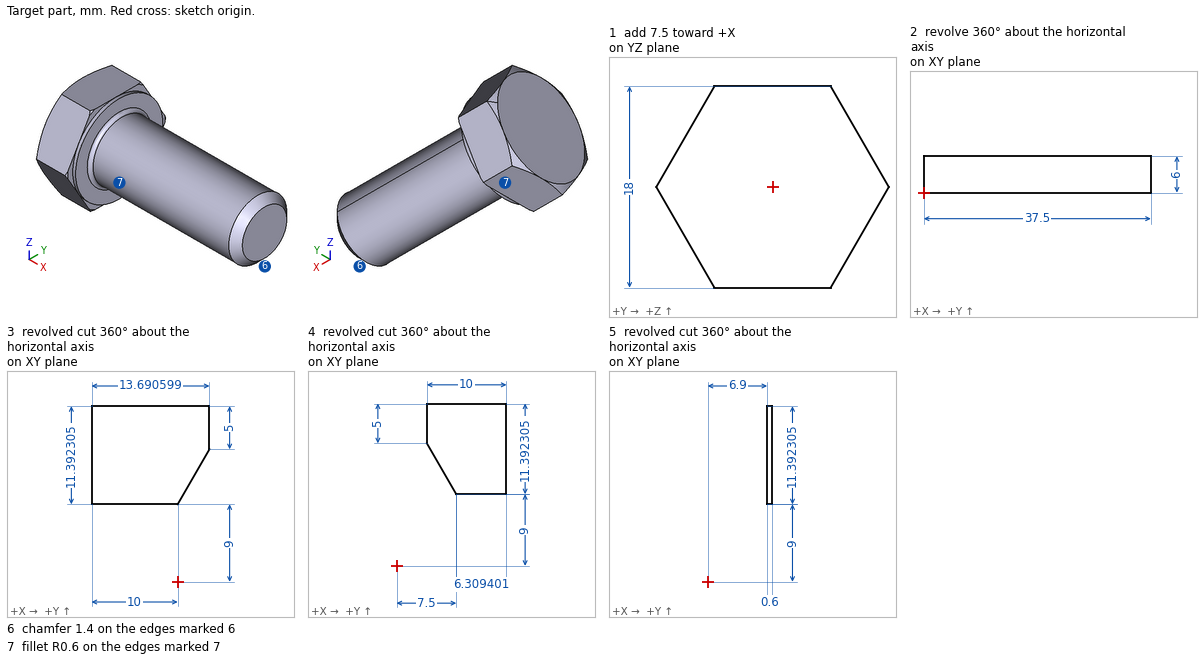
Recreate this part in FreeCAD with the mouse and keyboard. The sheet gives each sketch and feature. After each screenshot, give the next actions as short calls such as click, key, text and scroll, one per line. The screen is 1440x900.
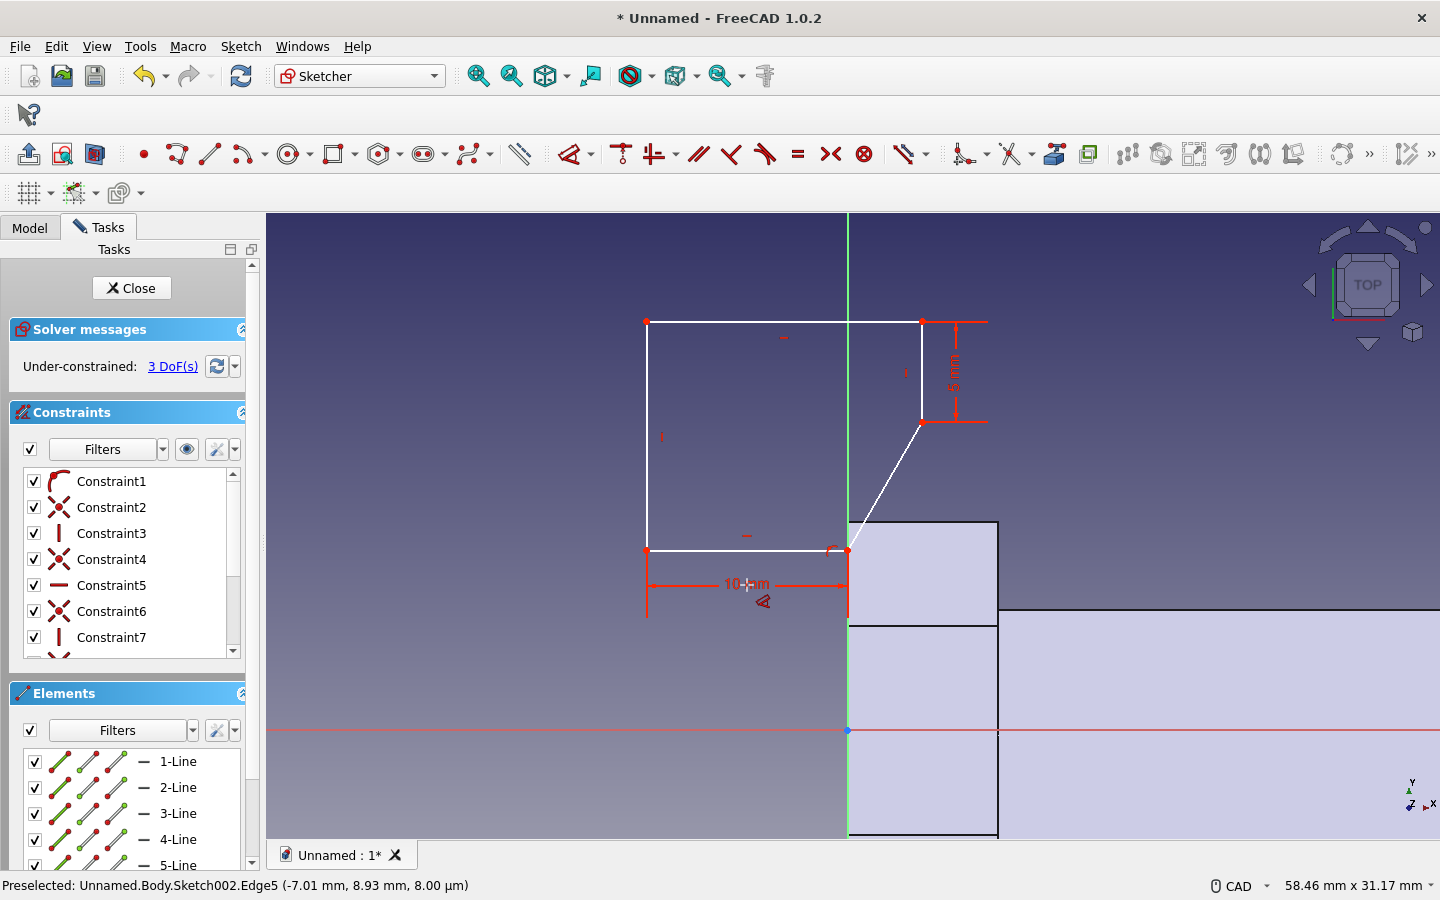
click(848, 551)
click(882, 641)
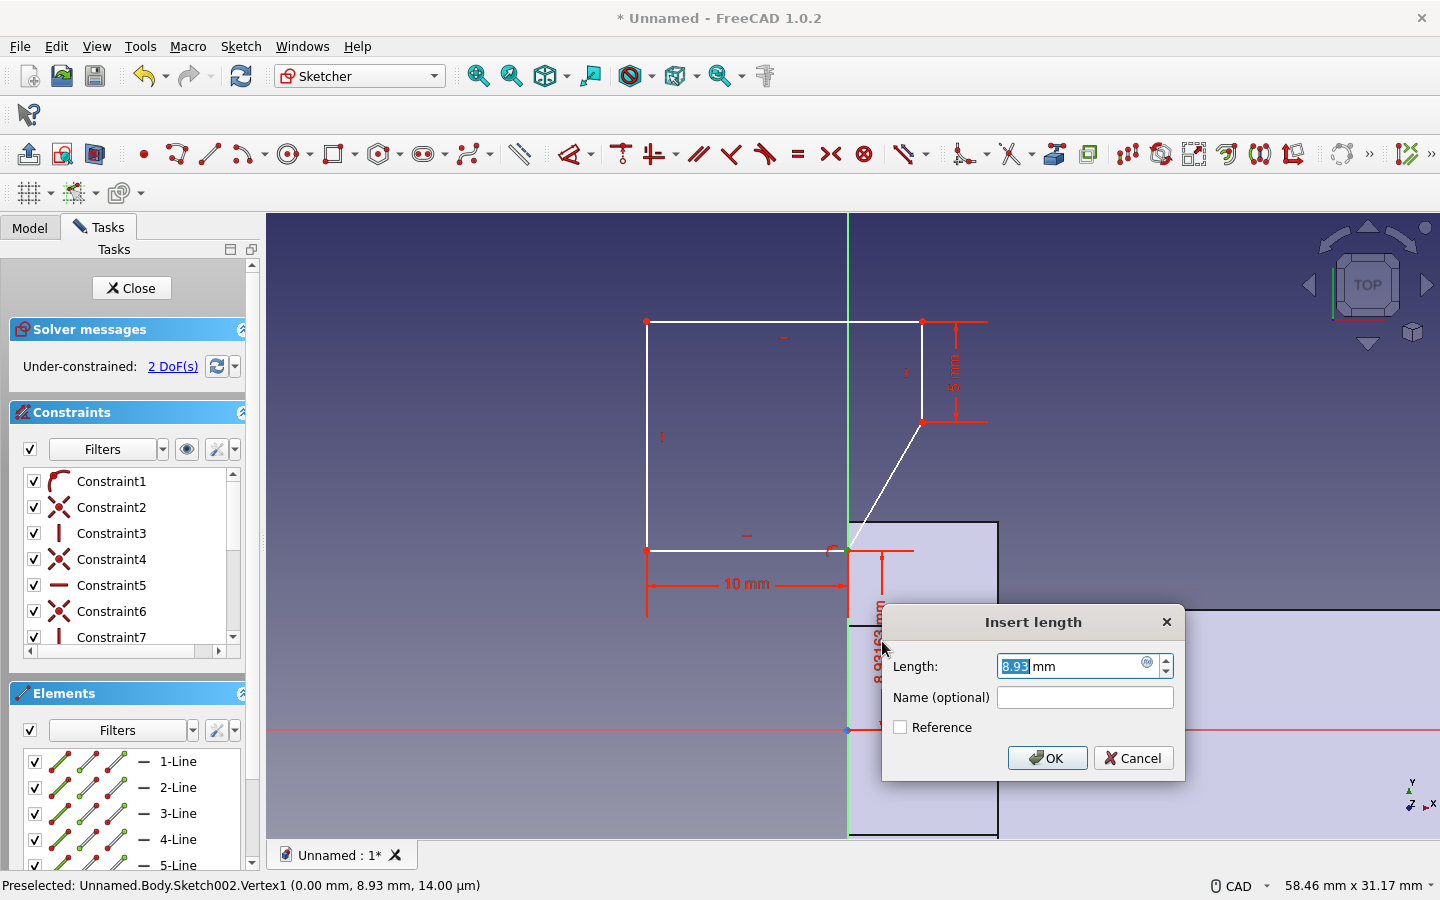
text(9)
key(Return)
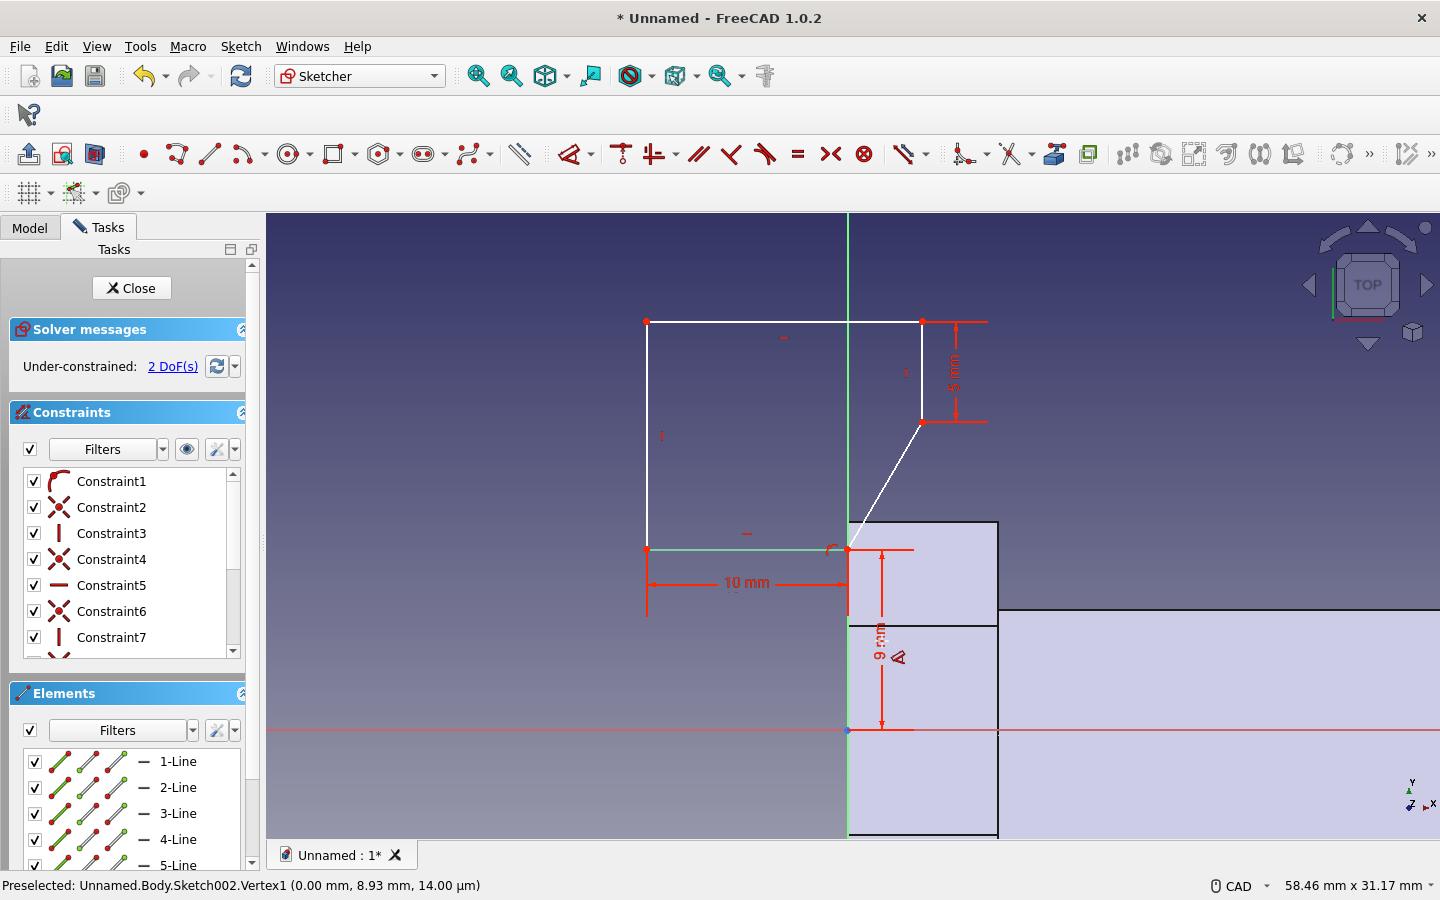
click(729, 322)
click(784, 288)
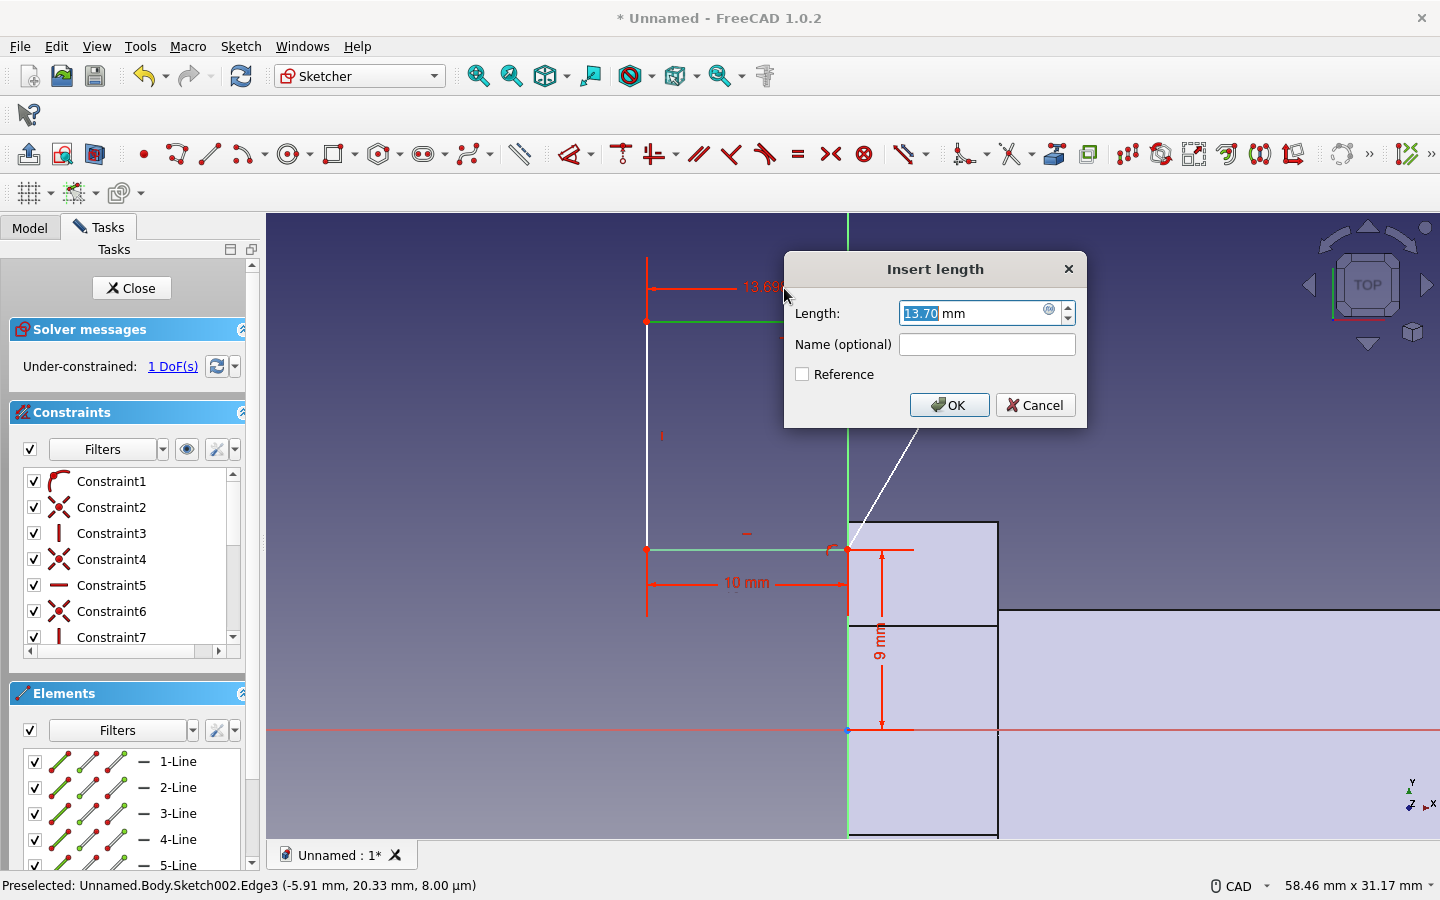
text(13.690599)
key(Return)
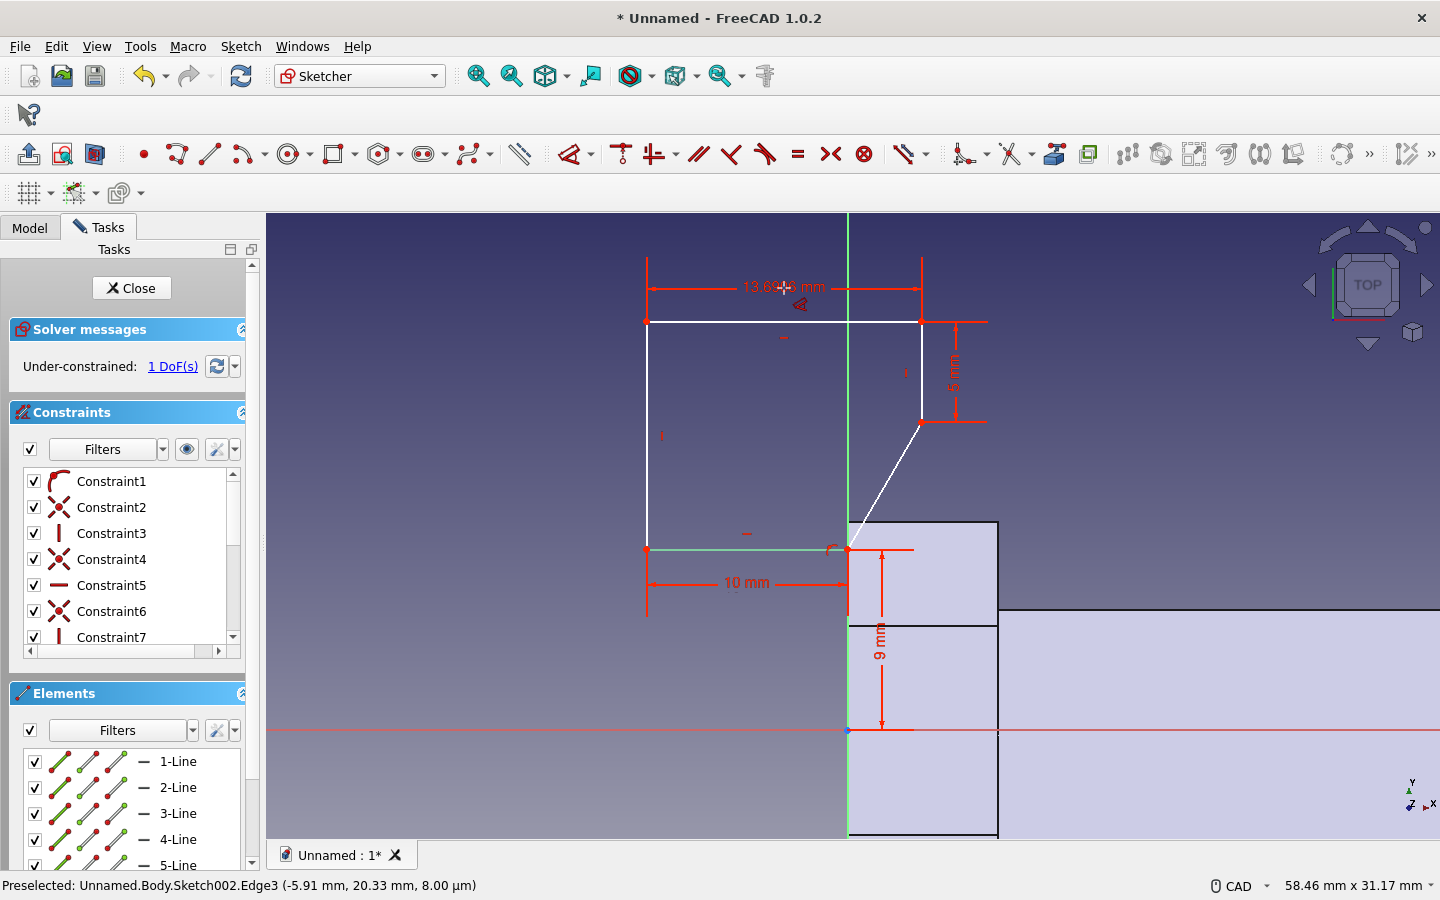
click(647, 390)
click(613, 436)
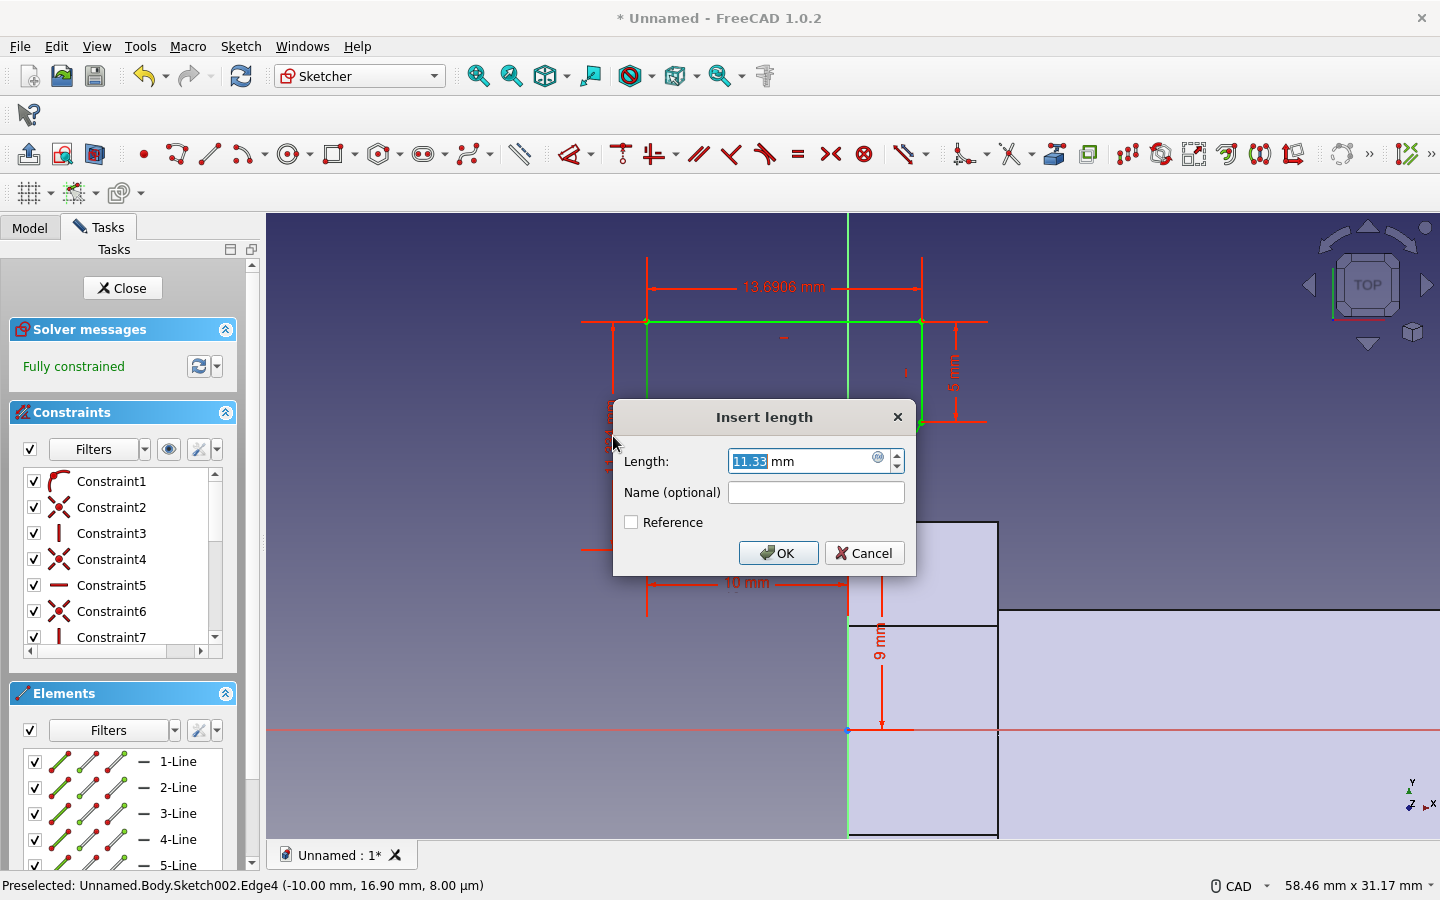
text(11.392305)
key(Return)
key(Escape)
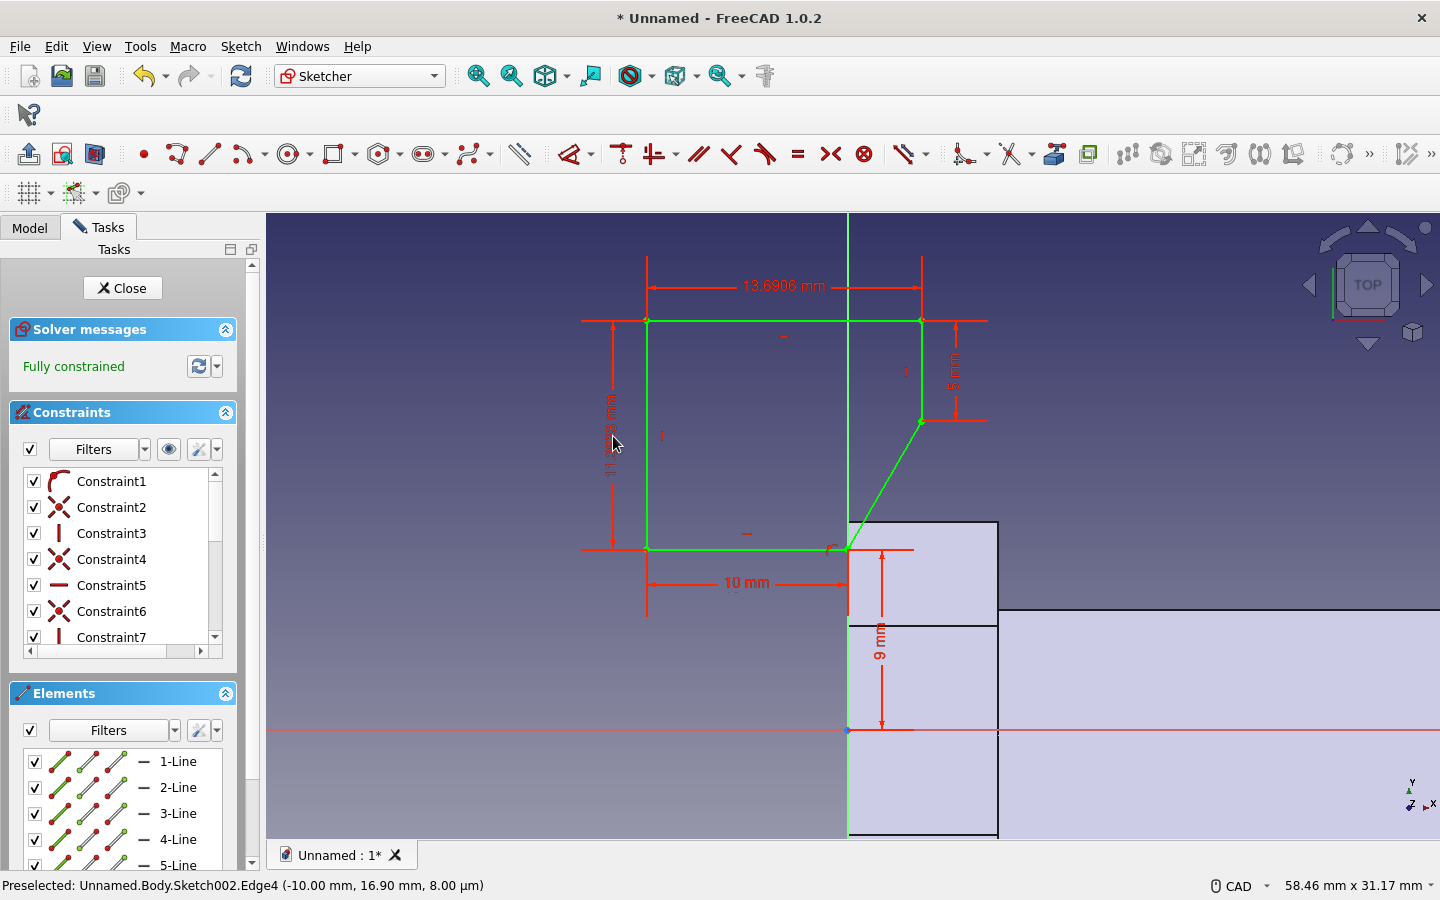
click(123, 288)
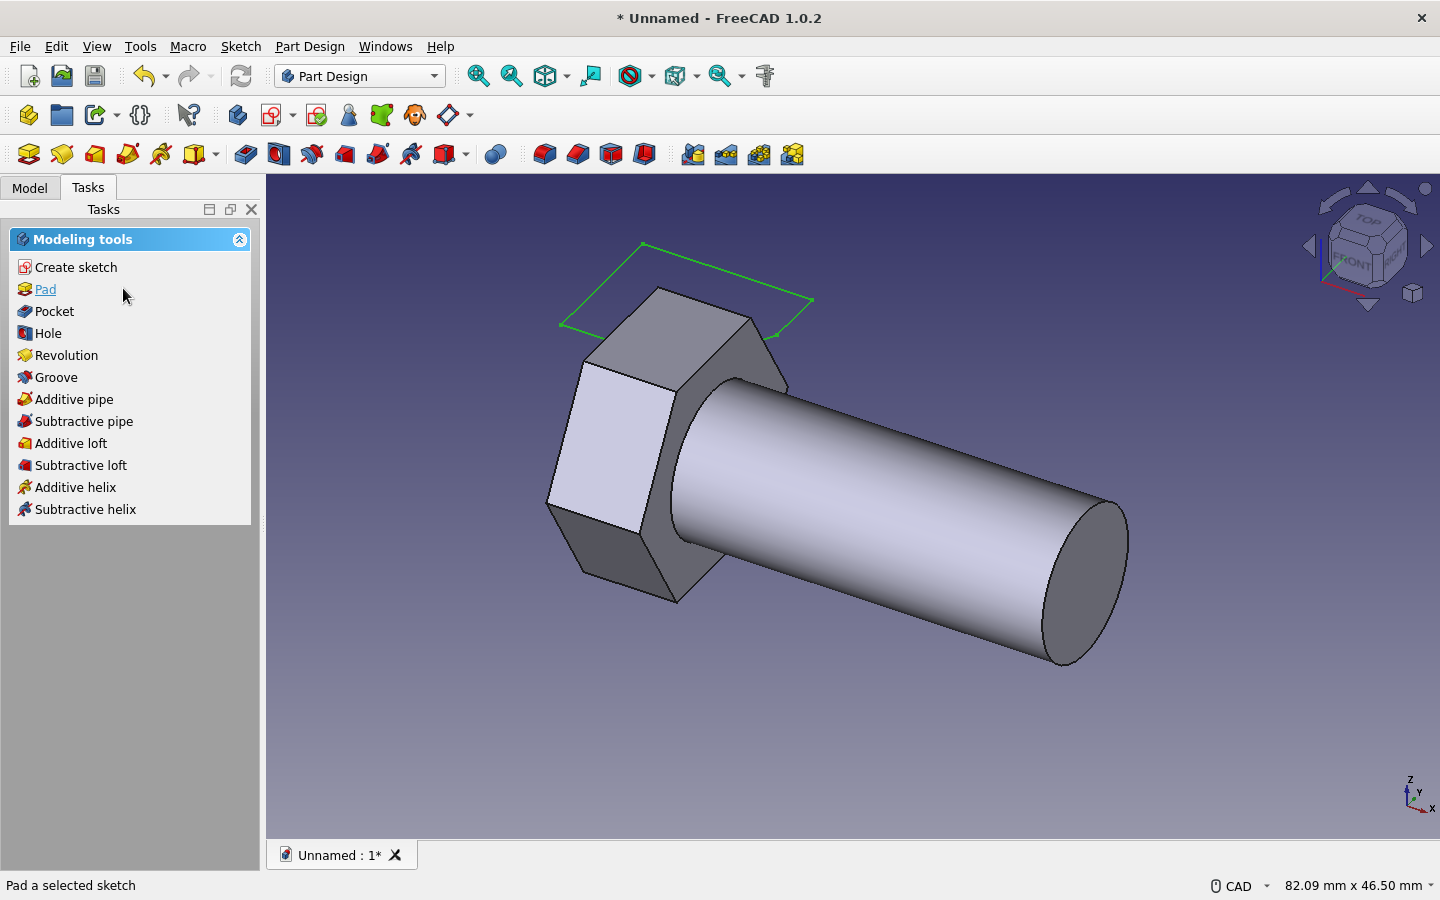
click(312, 154)